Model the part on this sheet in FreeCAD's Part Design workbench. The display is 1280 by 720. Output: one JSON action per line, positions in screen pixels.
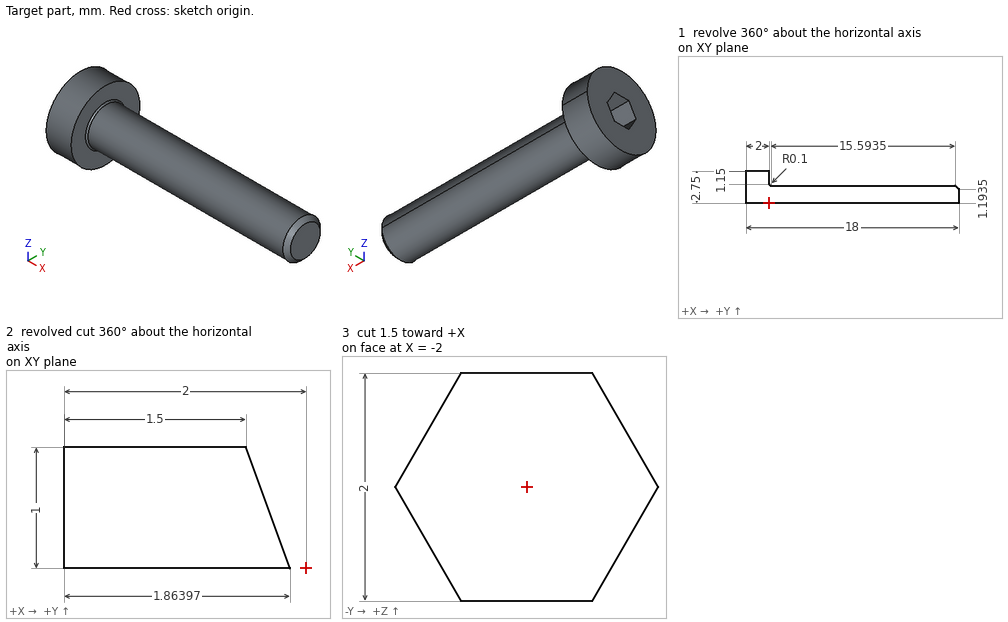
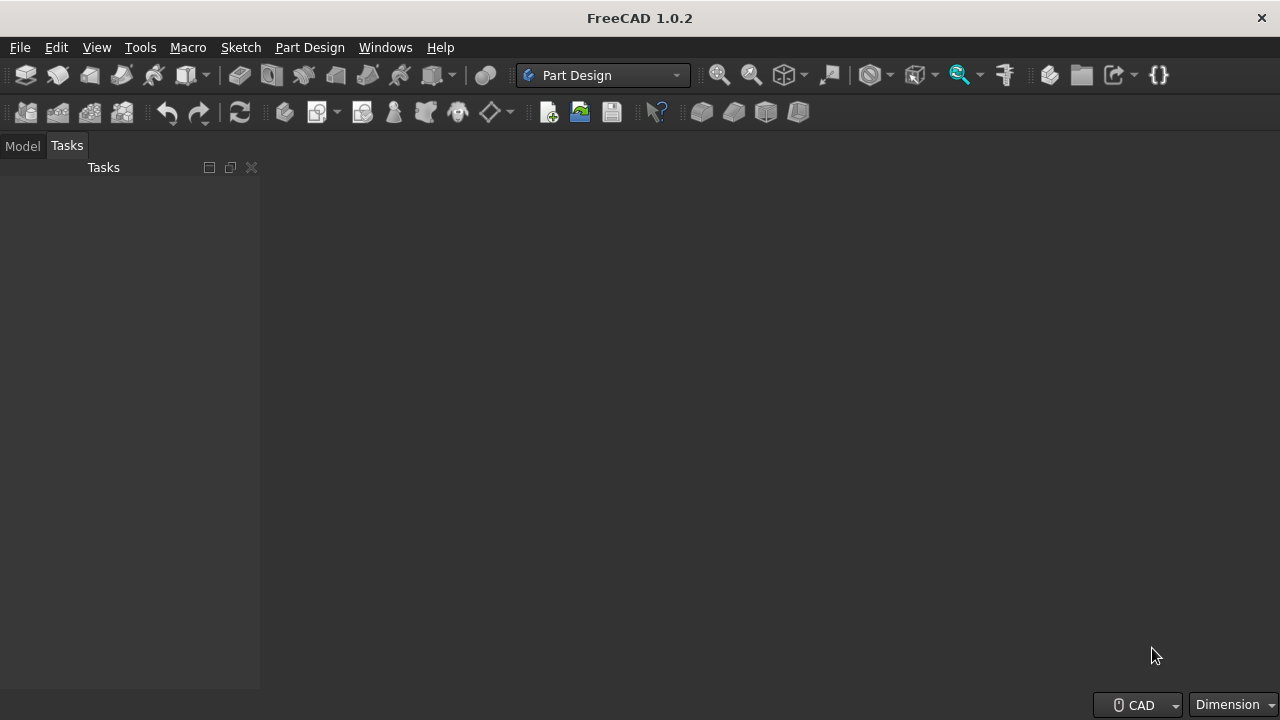
{"action": "left_click", "coordinate": [548, 112]}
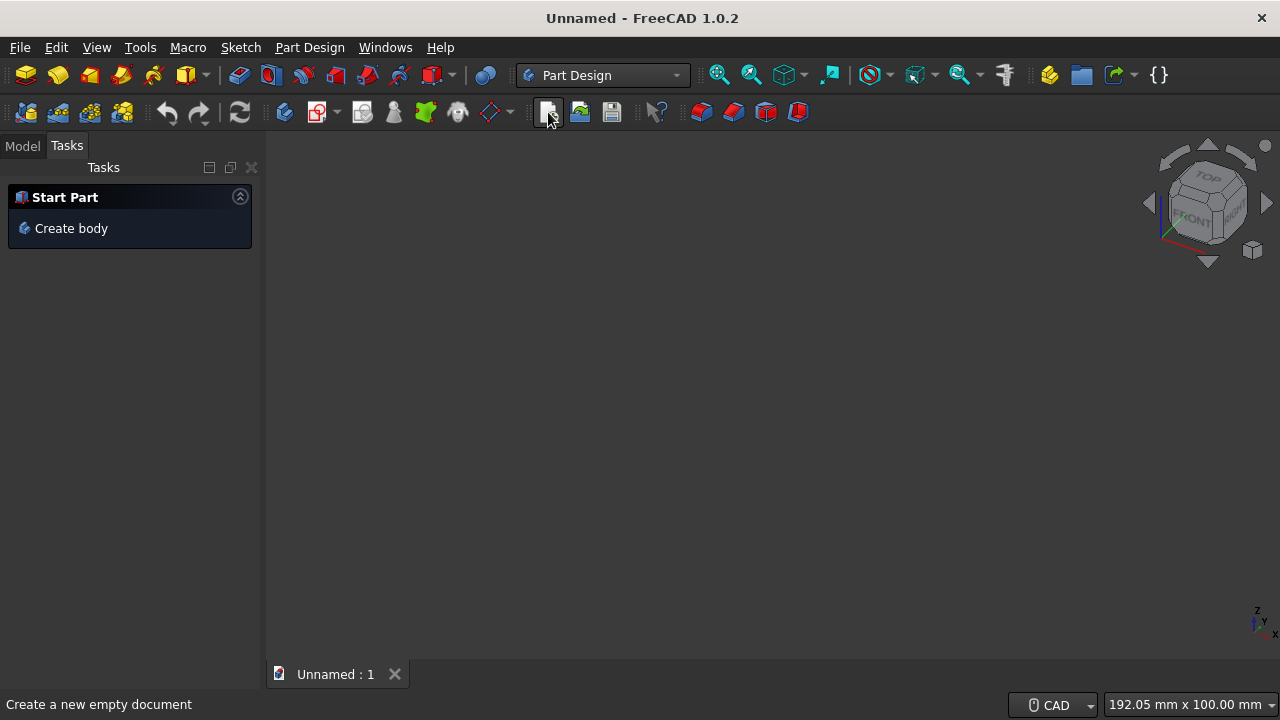
{"action": "left_click", "coordinate": [318, 112]}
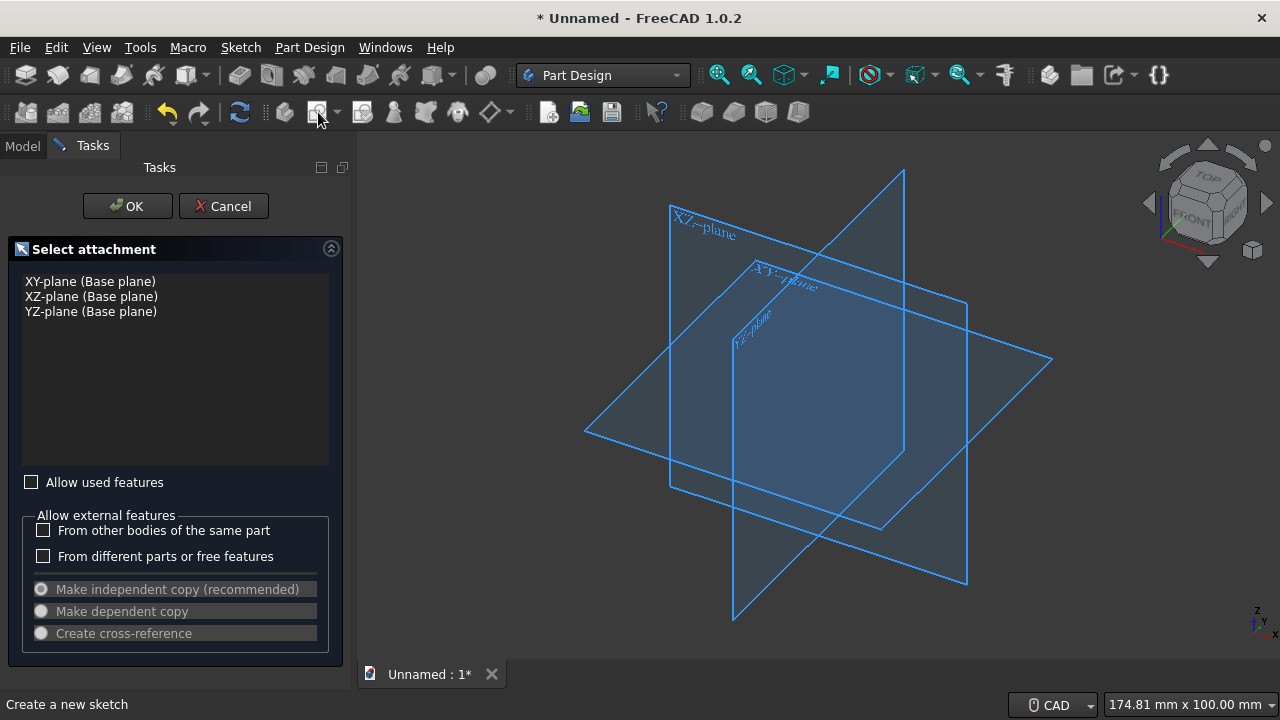
{"action": "left_click", "coordinate": [82, 282]}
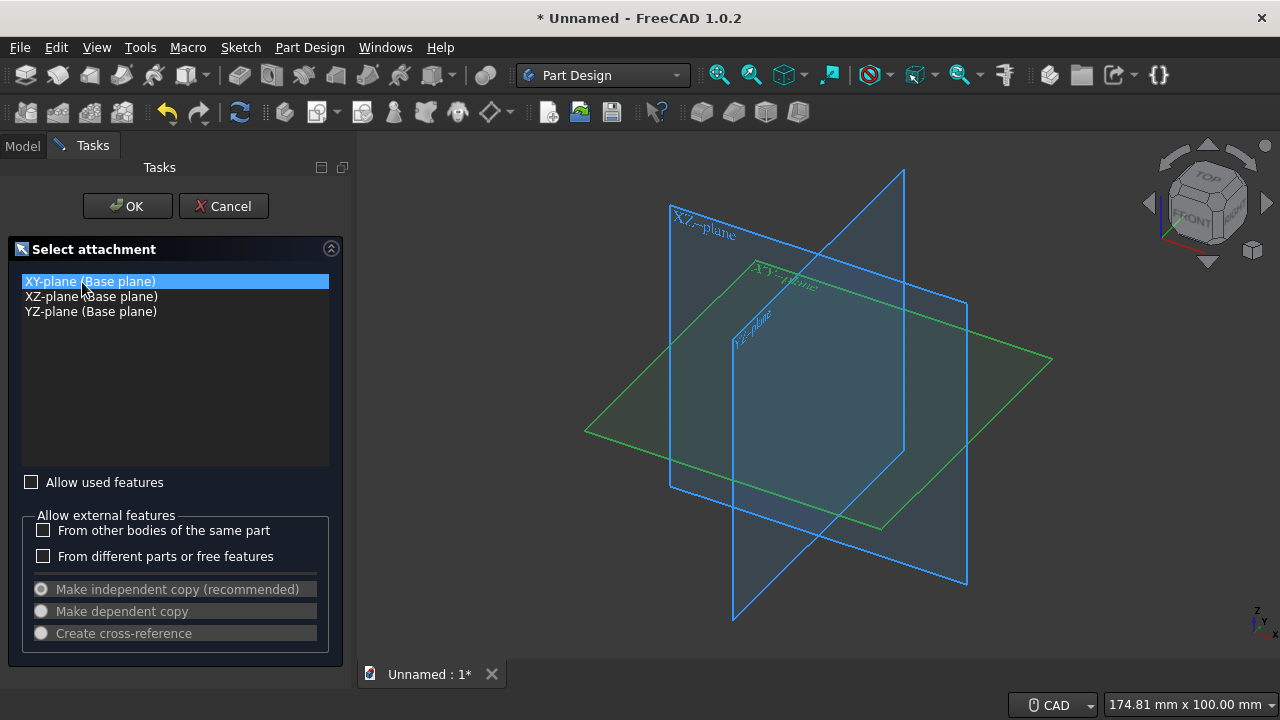
{"action": "left_click", "coordinate": [128, 206]}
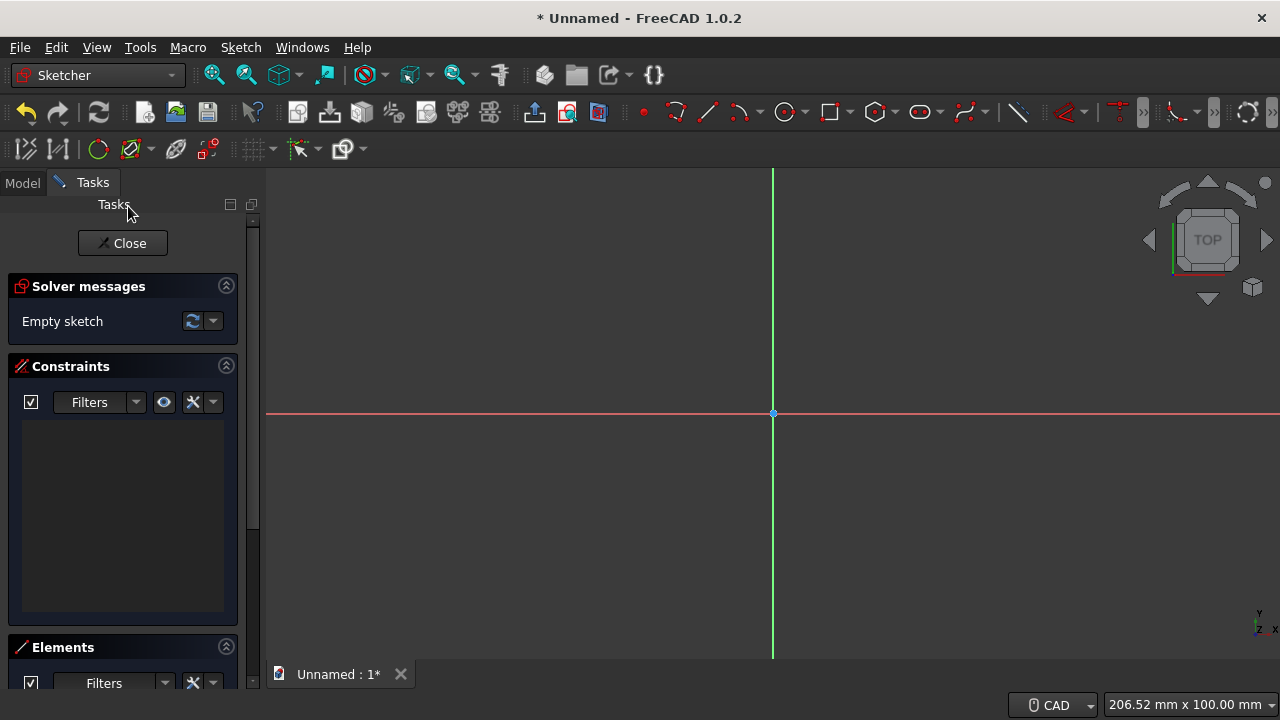
{"action": "scroll", "coordinate": [828, 405], "scroll_direction": "up", "scroll_amount": 9}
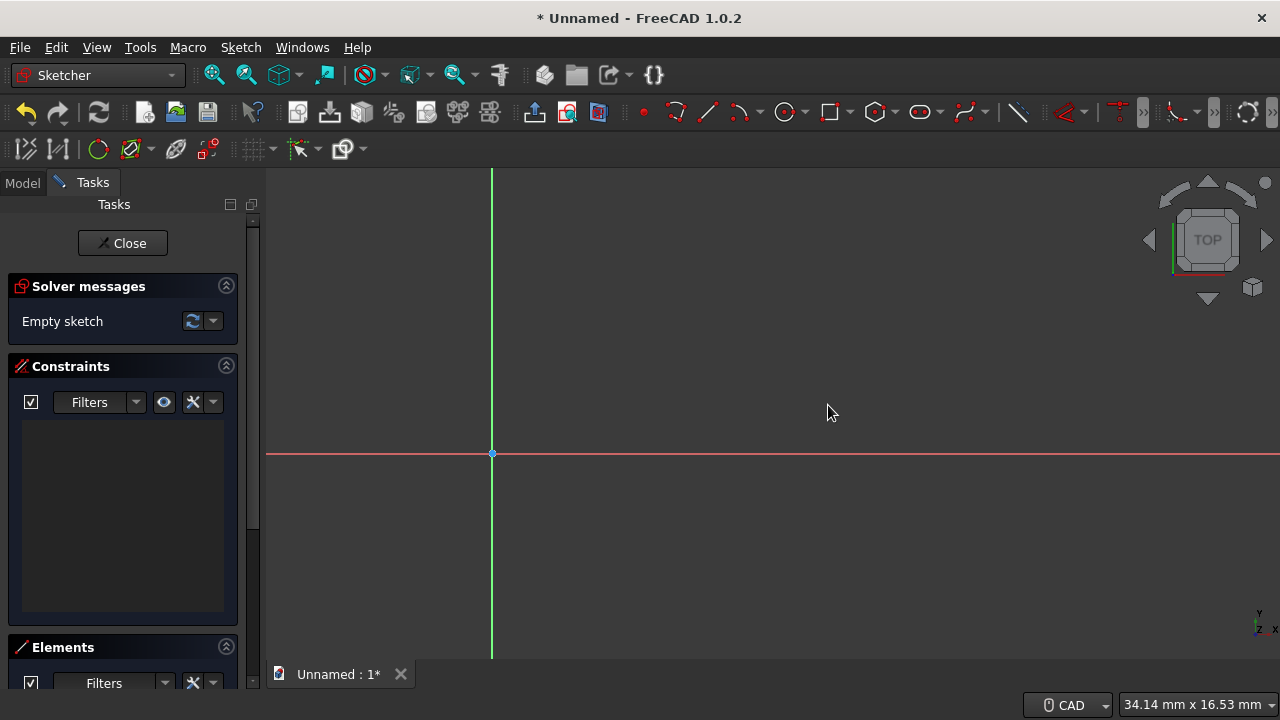
{"action": "left_click", "coordinate": [676, 112]}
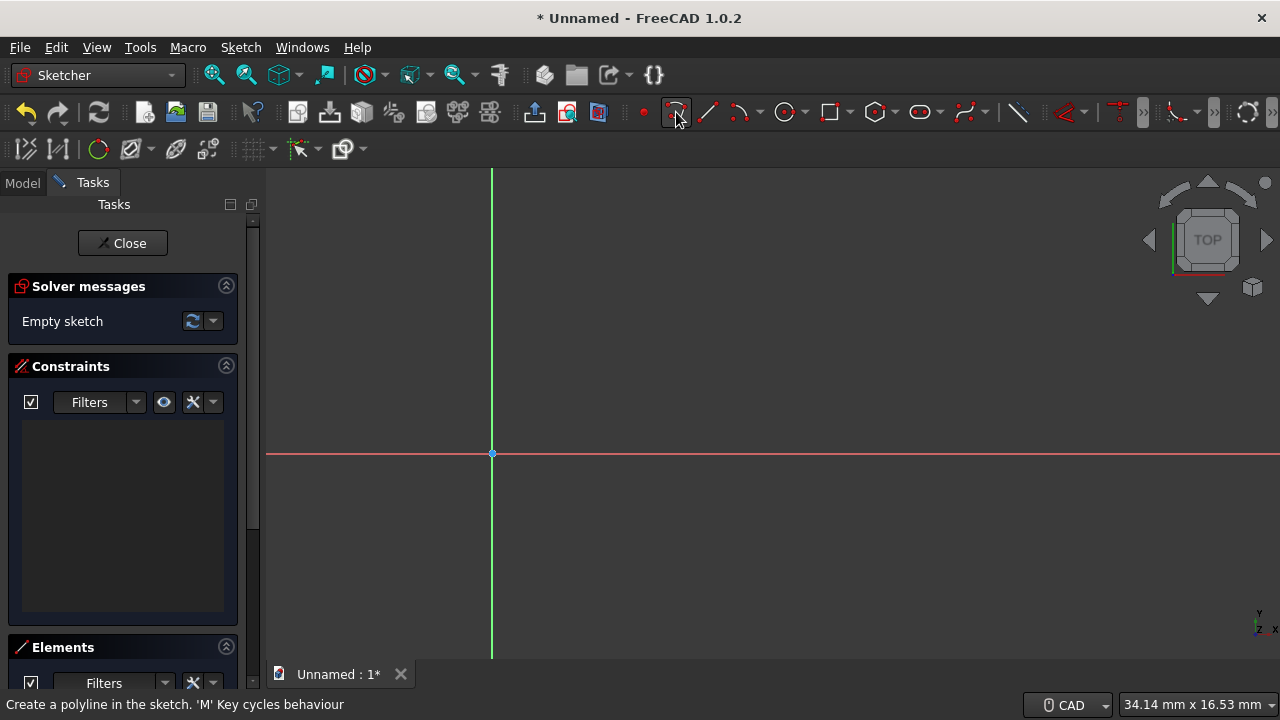
{"action": "left_click", "coordinate": [492, 406]}
{"action": "left_click", "coordinate": [501, 372]}
{"action": "left_click", "coordinate": [433, 372]}
{"action": "left_click", "coordinate": [433, 454]}
{"action": "left_click", "coordinate": [968, 445]}
{"action": "left_click", "coordinate": [968, 419]}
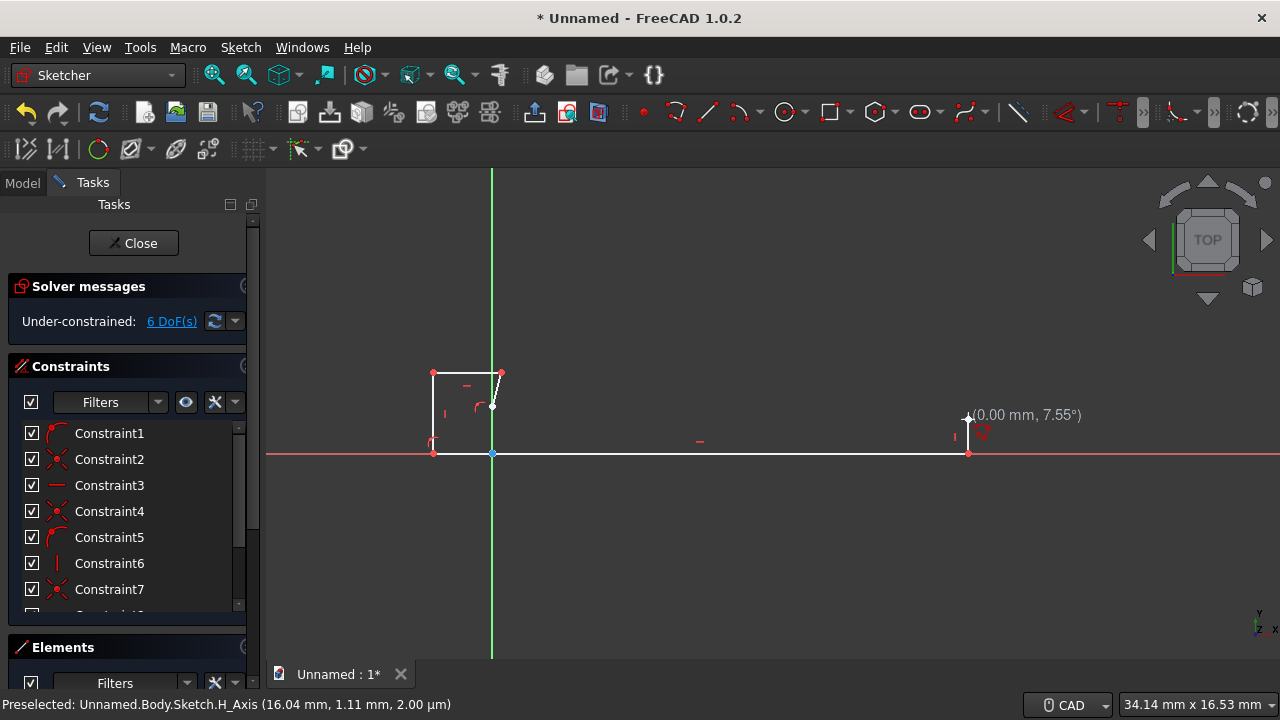
{"action": "scroll", "coordinate": [959, 409], "scroll_direction": "up", "scroll_amount": 2}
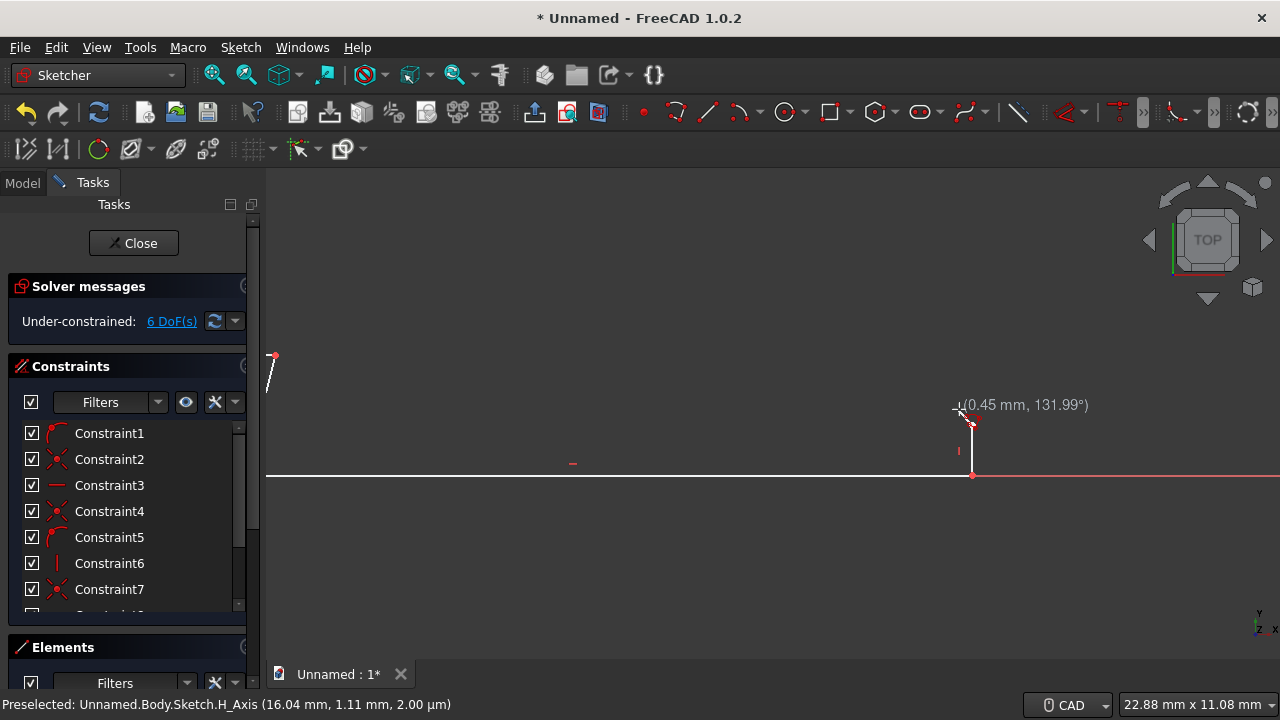
{"action": "left_click", "coordinate": [958, 409]}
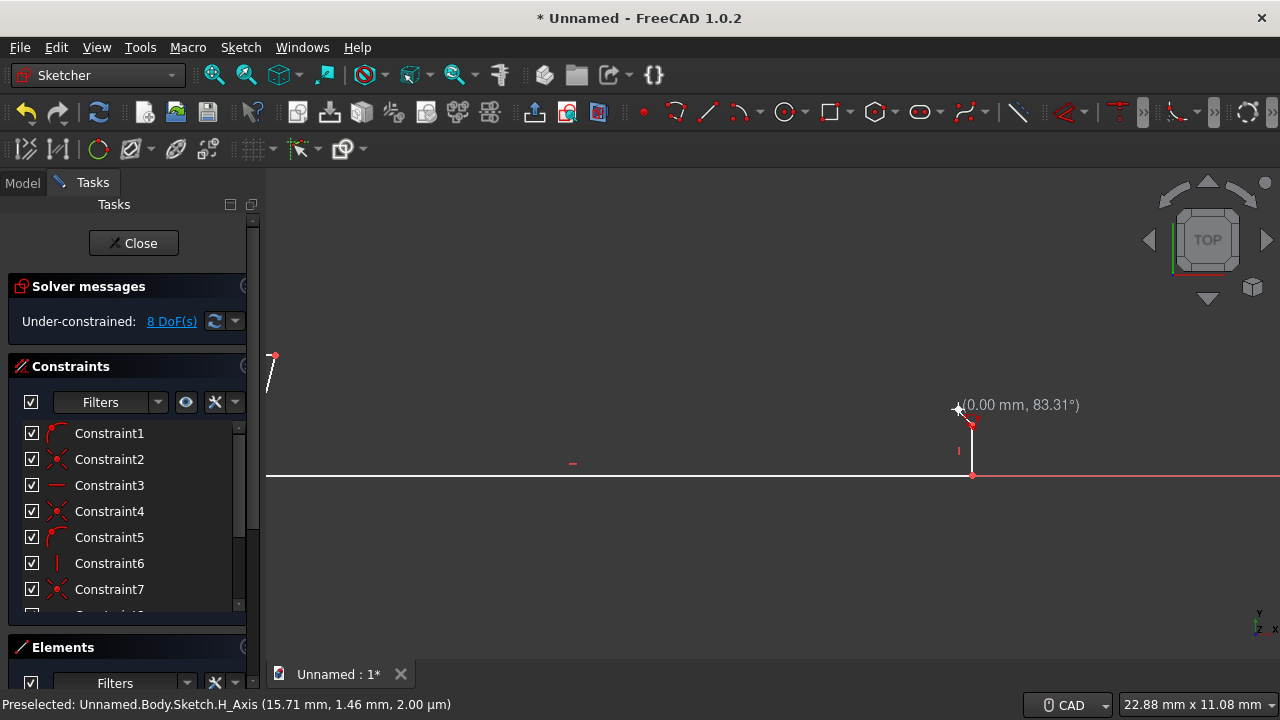
{"action": "scroll", "coordinate": [972, 411], "scroll_direction": "down", "scroll_amount": 2}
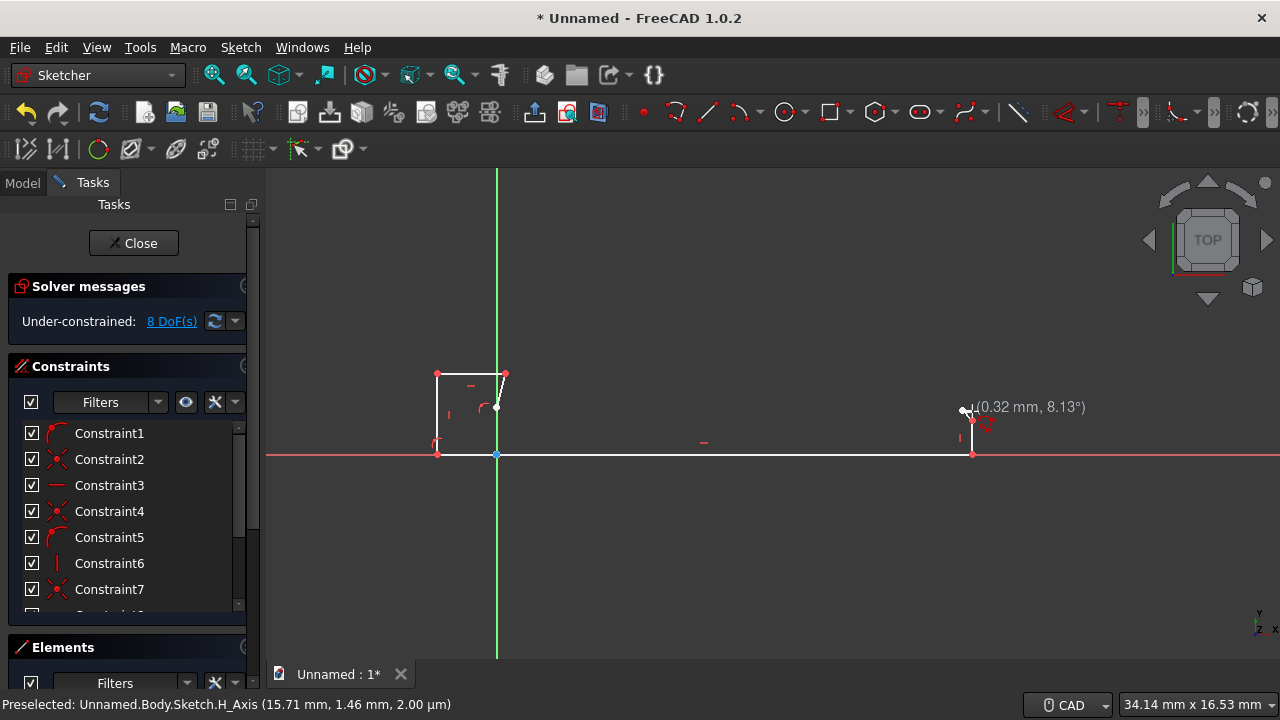
{"action": "scroll", "coordinate": [500, 410], "scroll_direction": "up", "scroll_amount": 9}